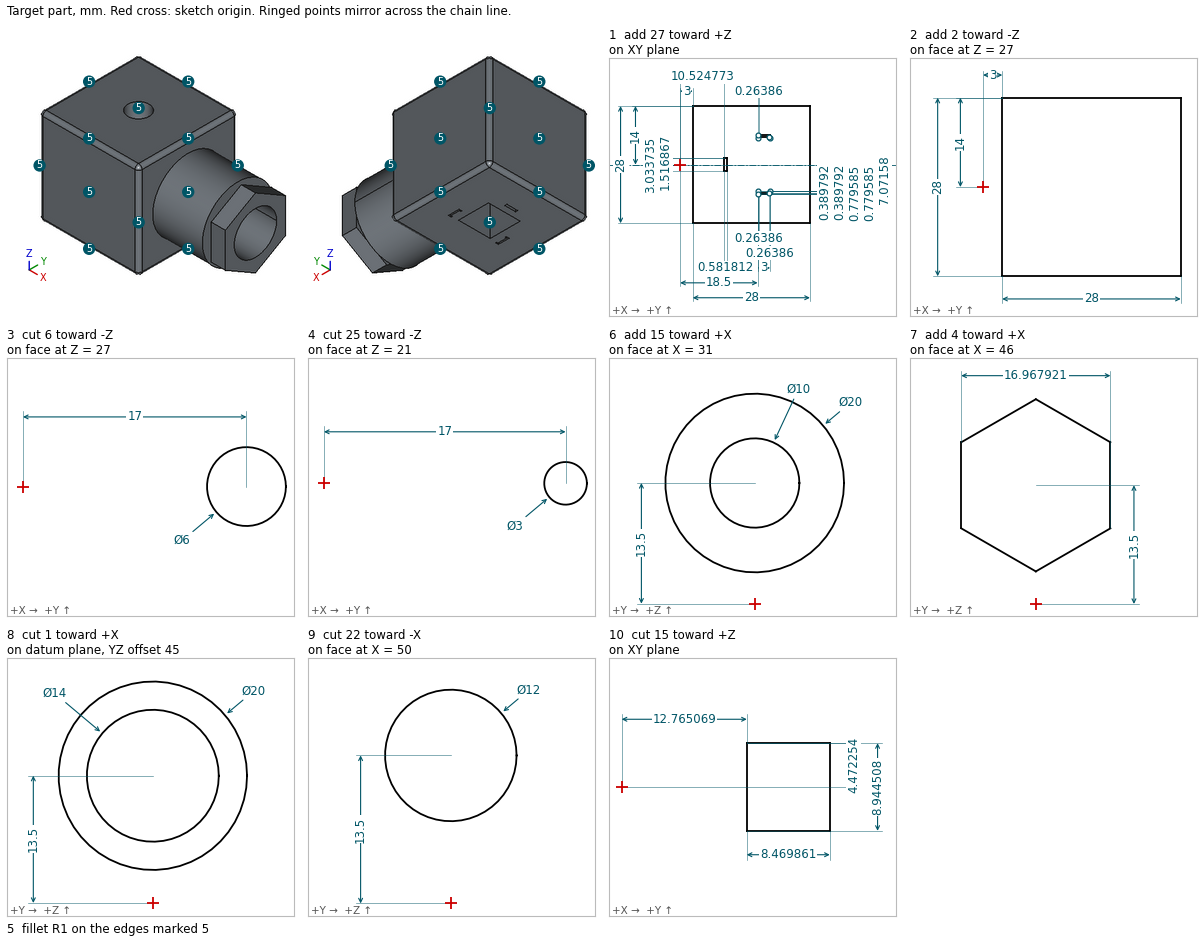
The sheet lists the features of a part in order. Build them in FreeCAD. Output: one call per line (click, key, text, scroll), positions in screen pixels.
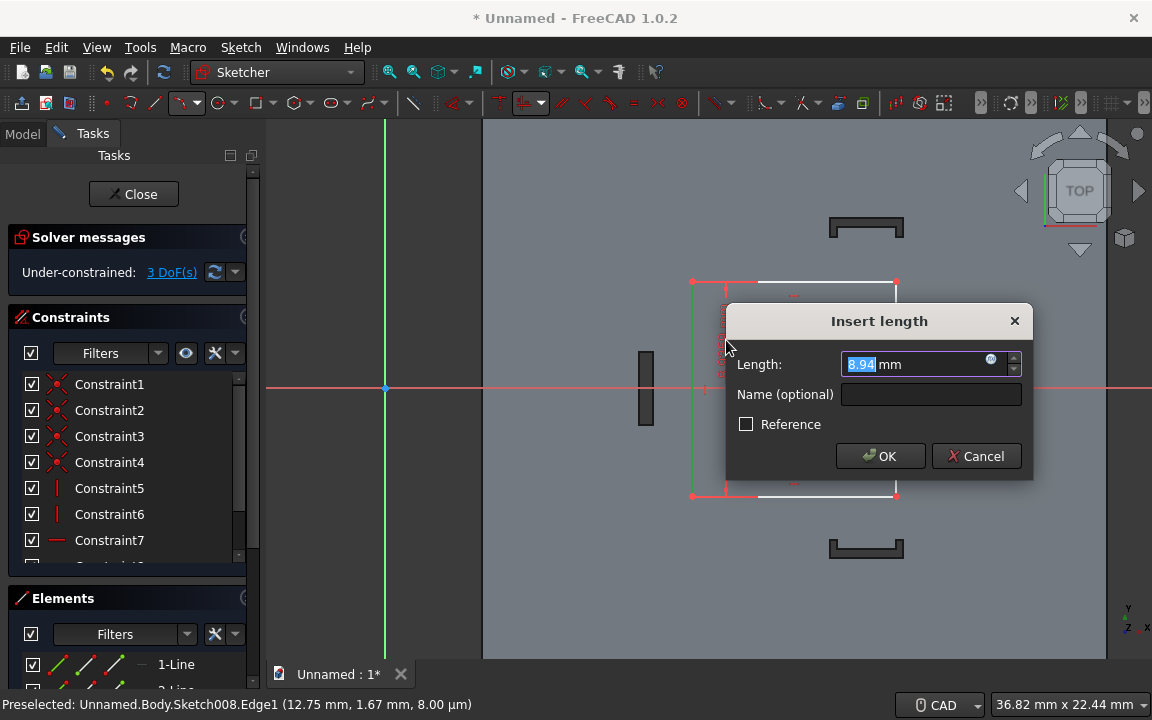
text(8.944508)
key(Return)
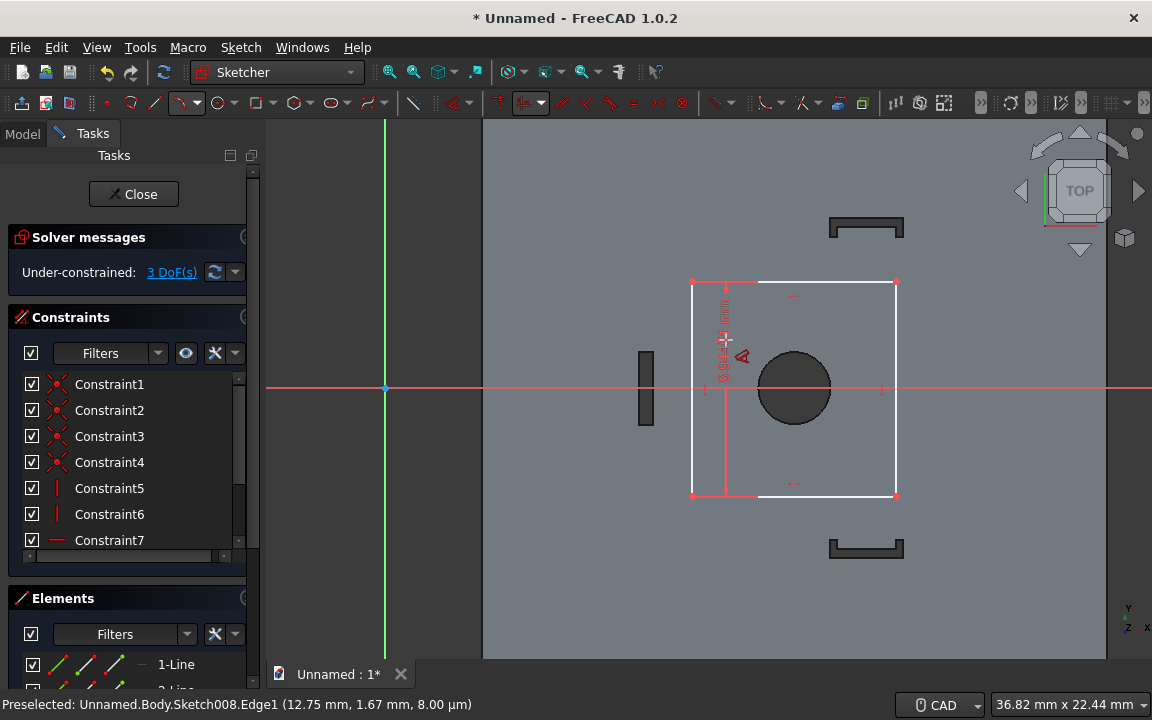
click(753, 497)
click(794, 531)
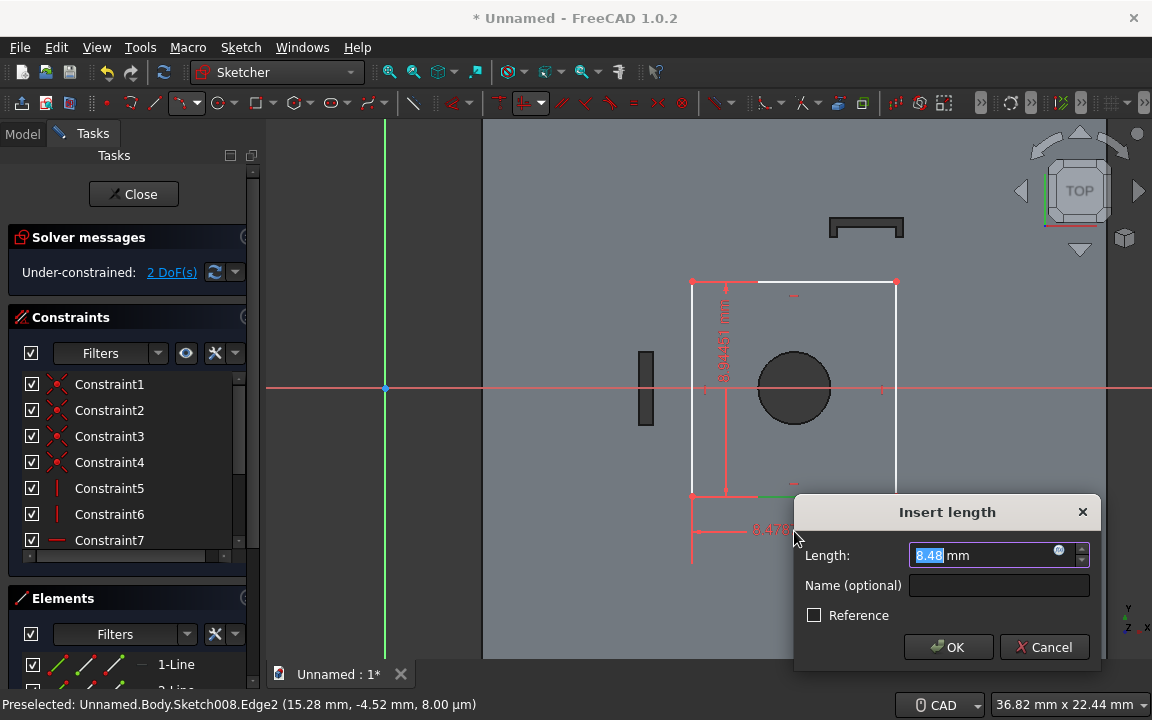
text(8.469861)
key(Return)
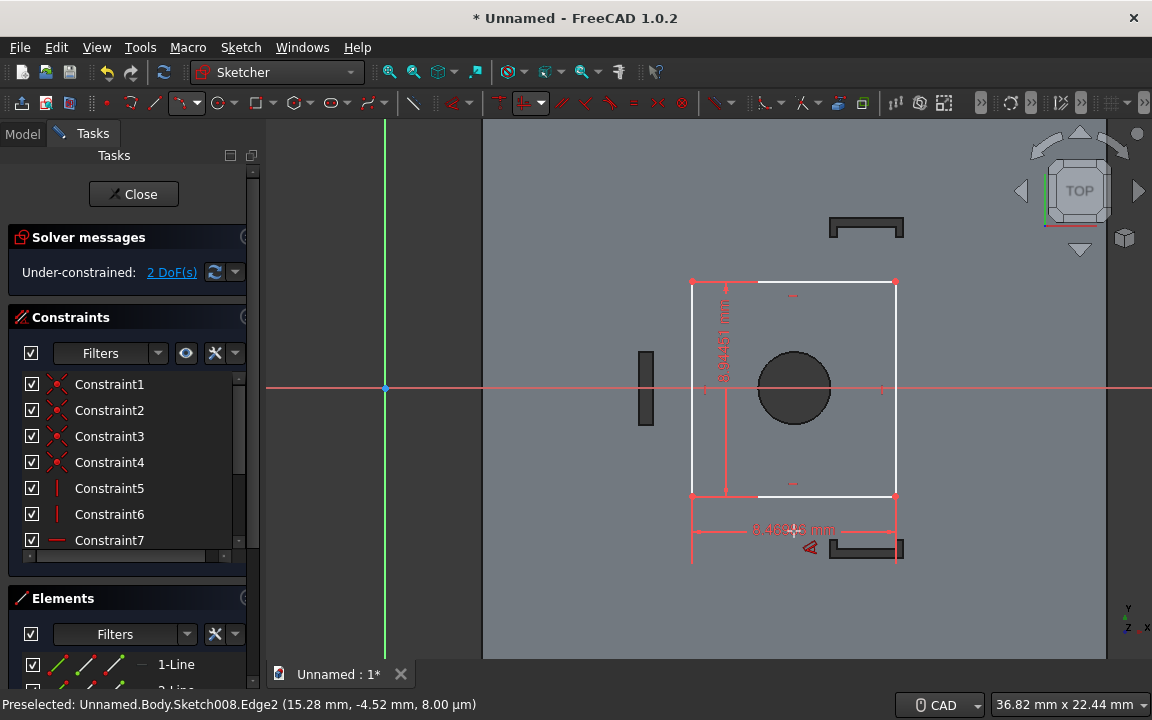
click(692, 282)
click(351, 335)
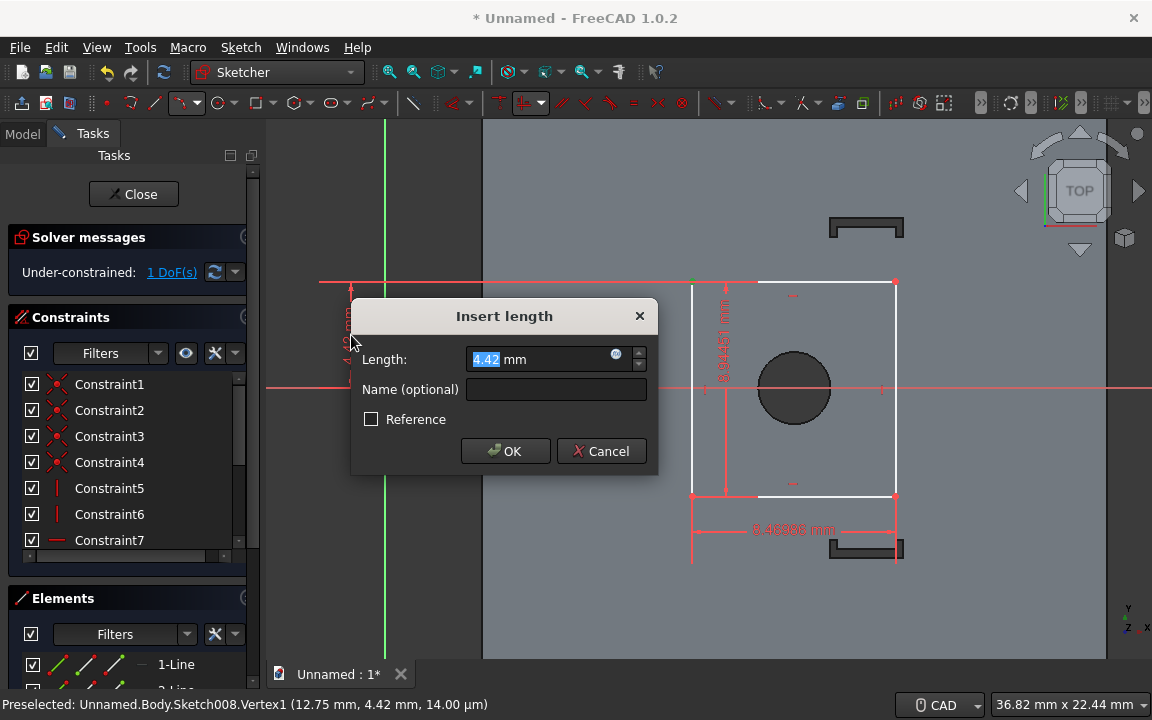
text(4.472254)
key(Return)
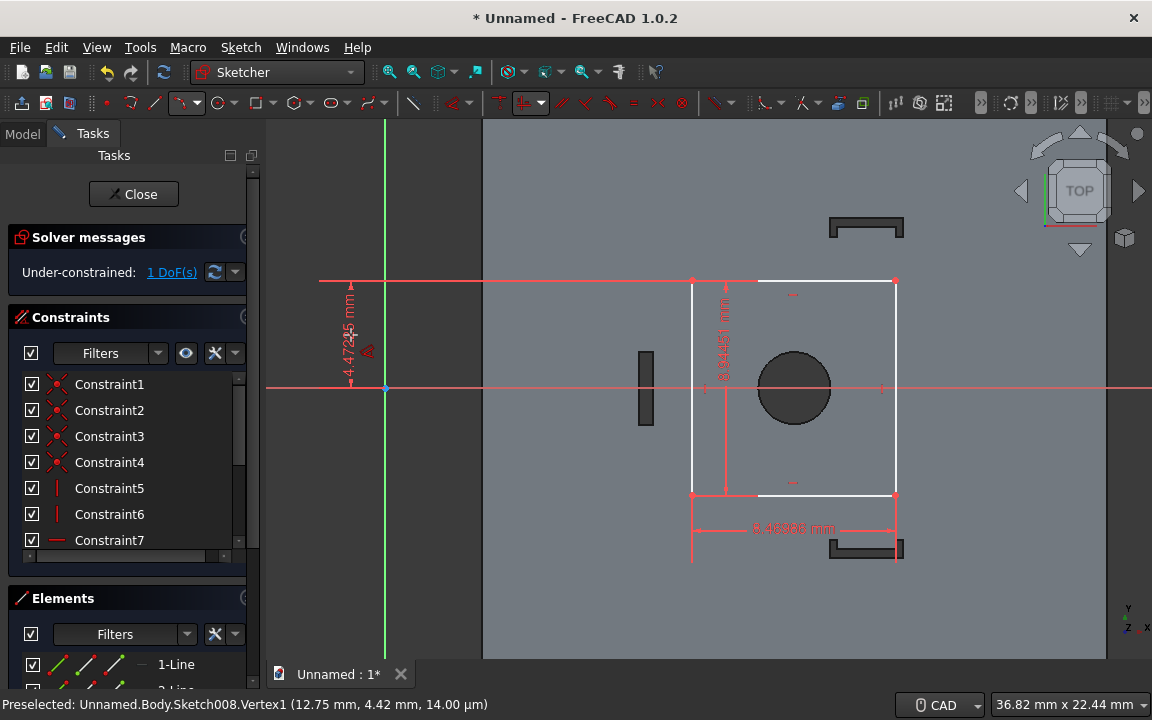
click(692, 281)
click(539, 247)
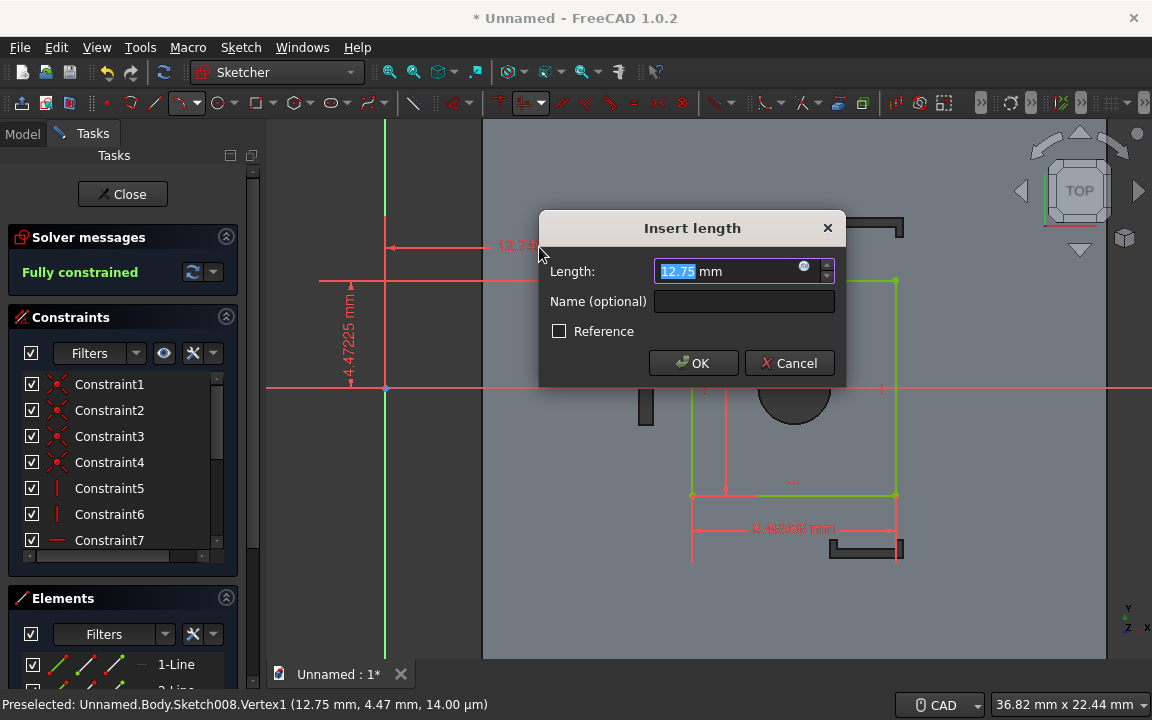
text(12.765069)
key(Return)
key(Escape)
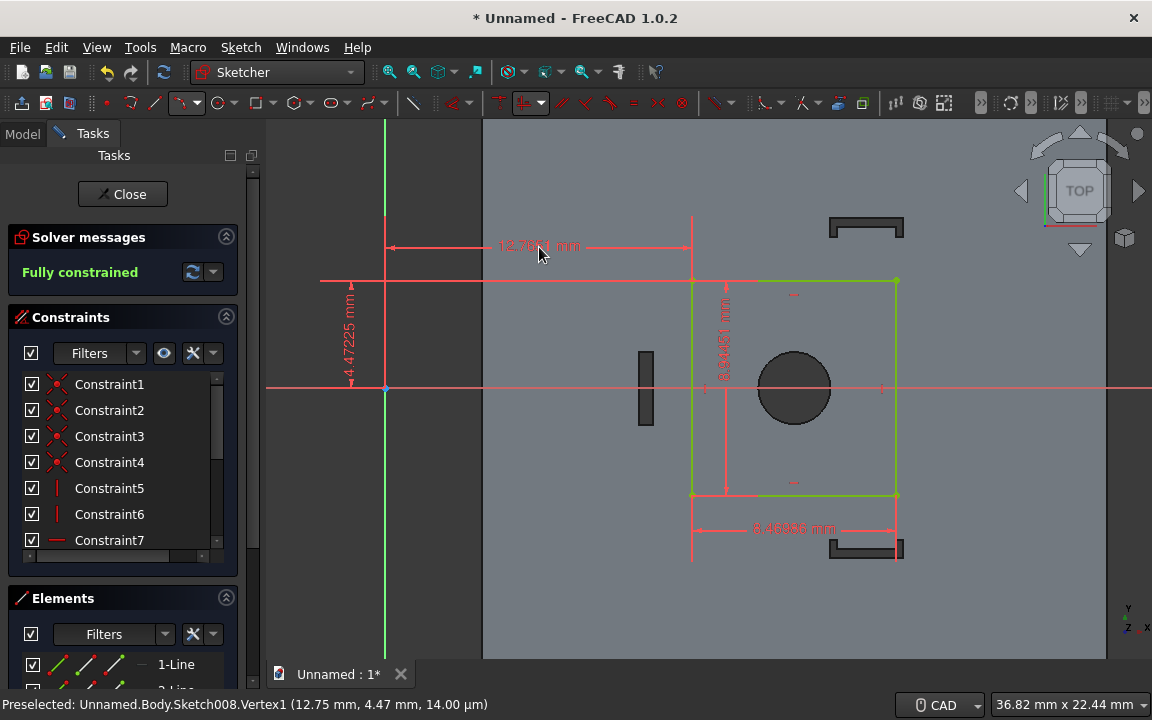
click(123, 194)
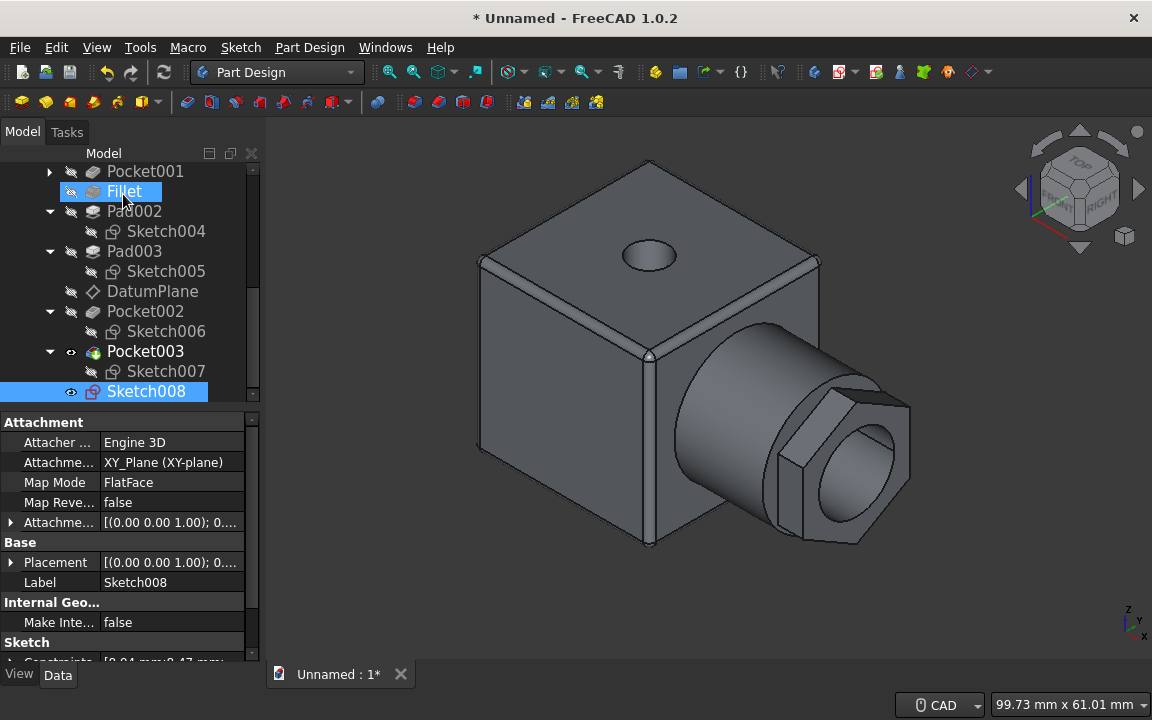
click(188, 102)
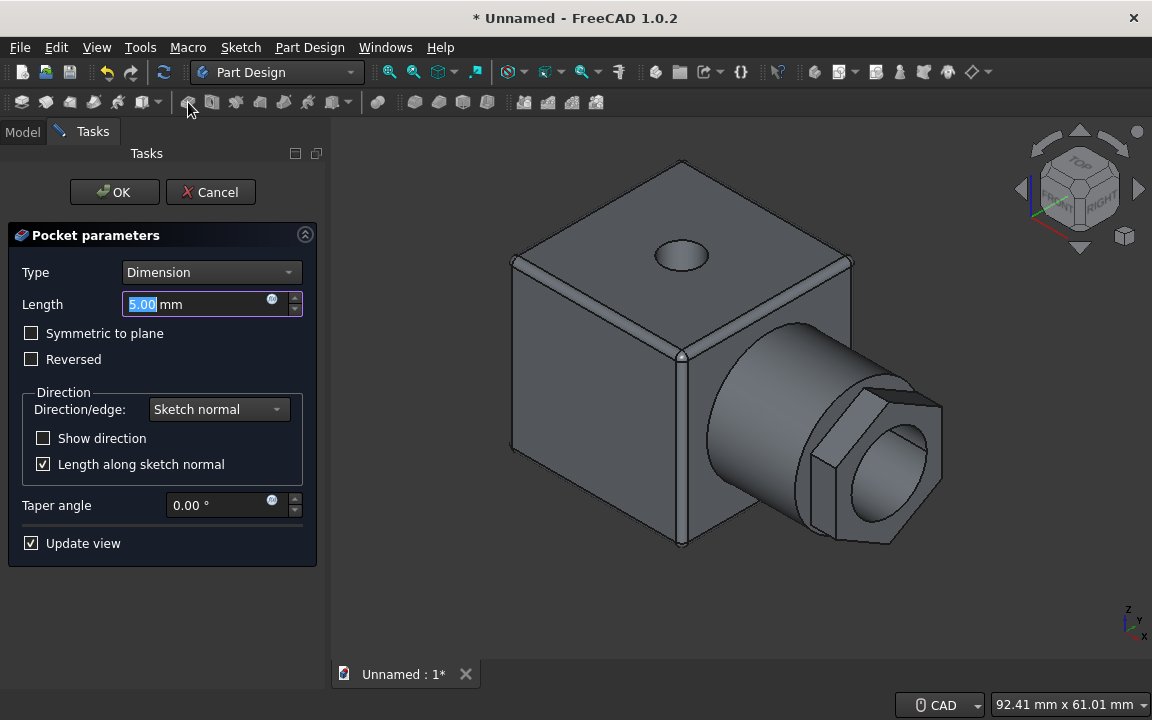
text(15)
key(Tab)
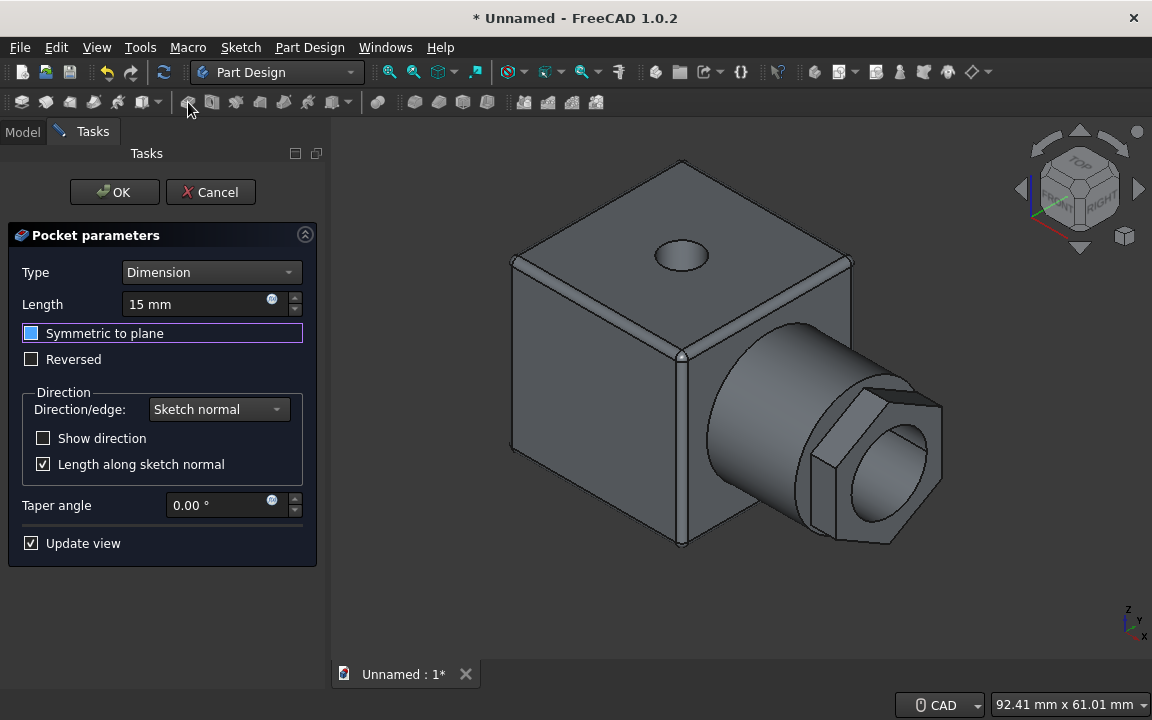
click(30, 359)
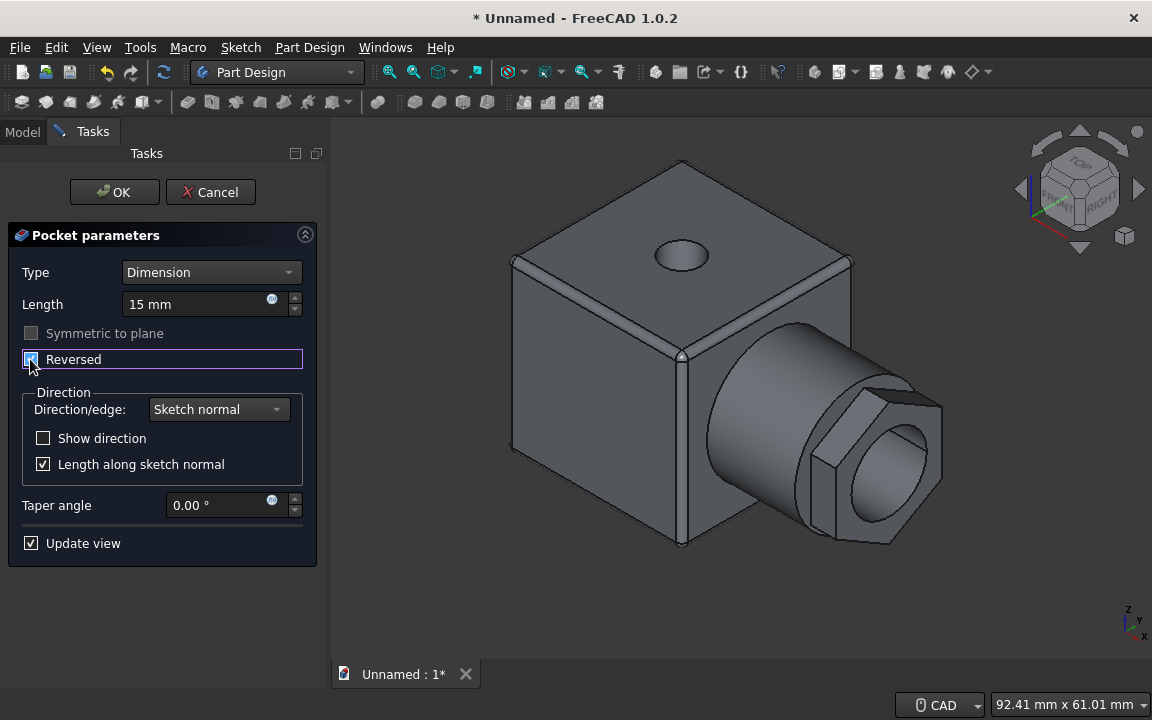
click(115, 192)